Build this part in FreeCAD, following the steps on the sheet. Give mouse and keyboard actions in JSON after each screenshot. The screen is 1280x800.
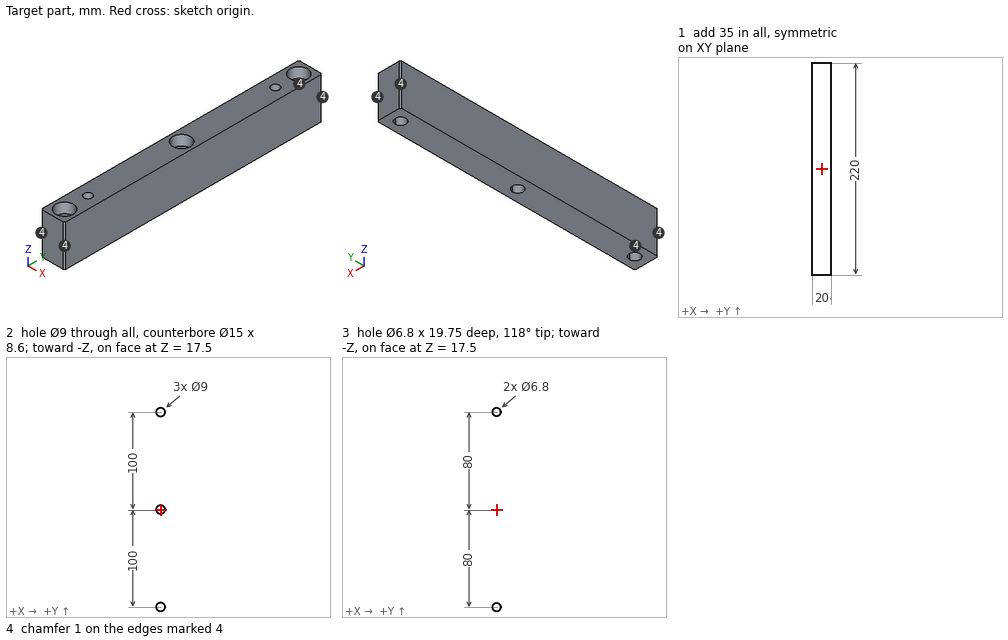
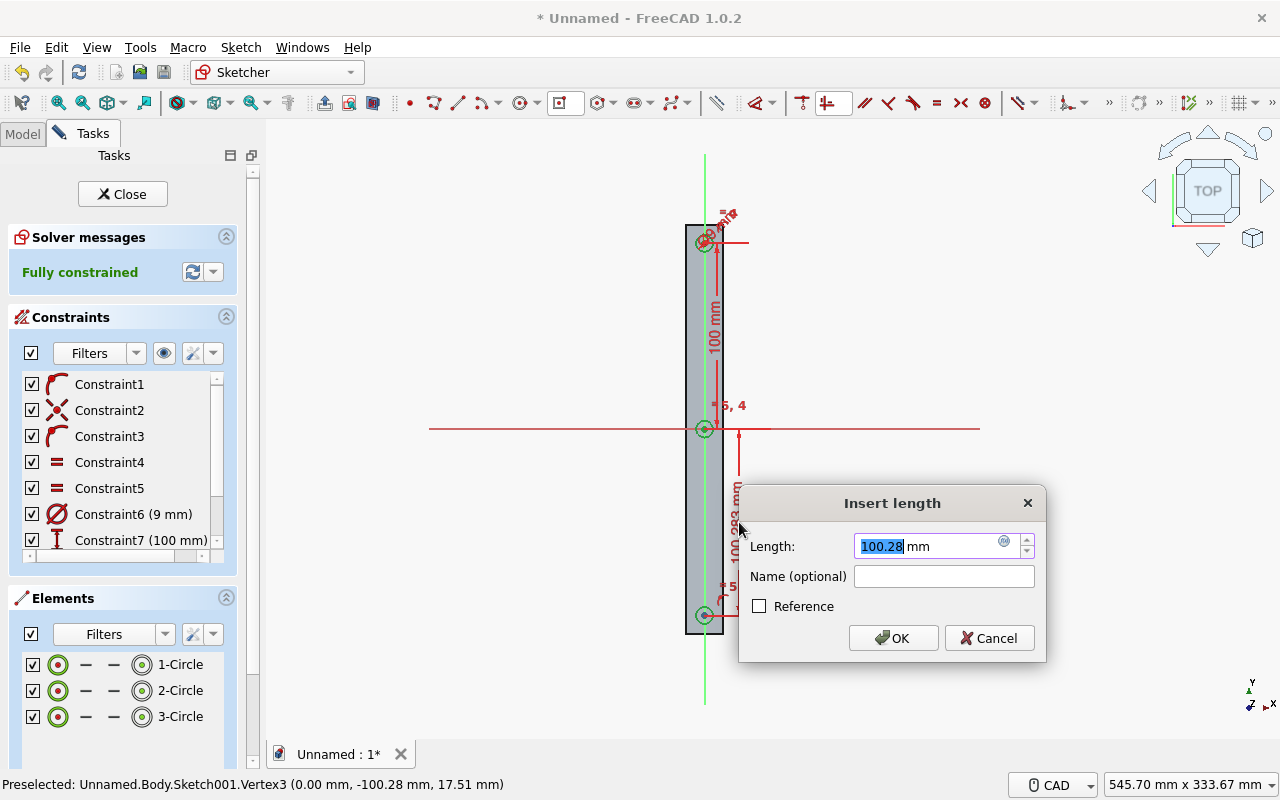
{"action": "type", "text": "100"}
{"action": "key", "text": "Return"}
{"action": "key", "text": "Escape"}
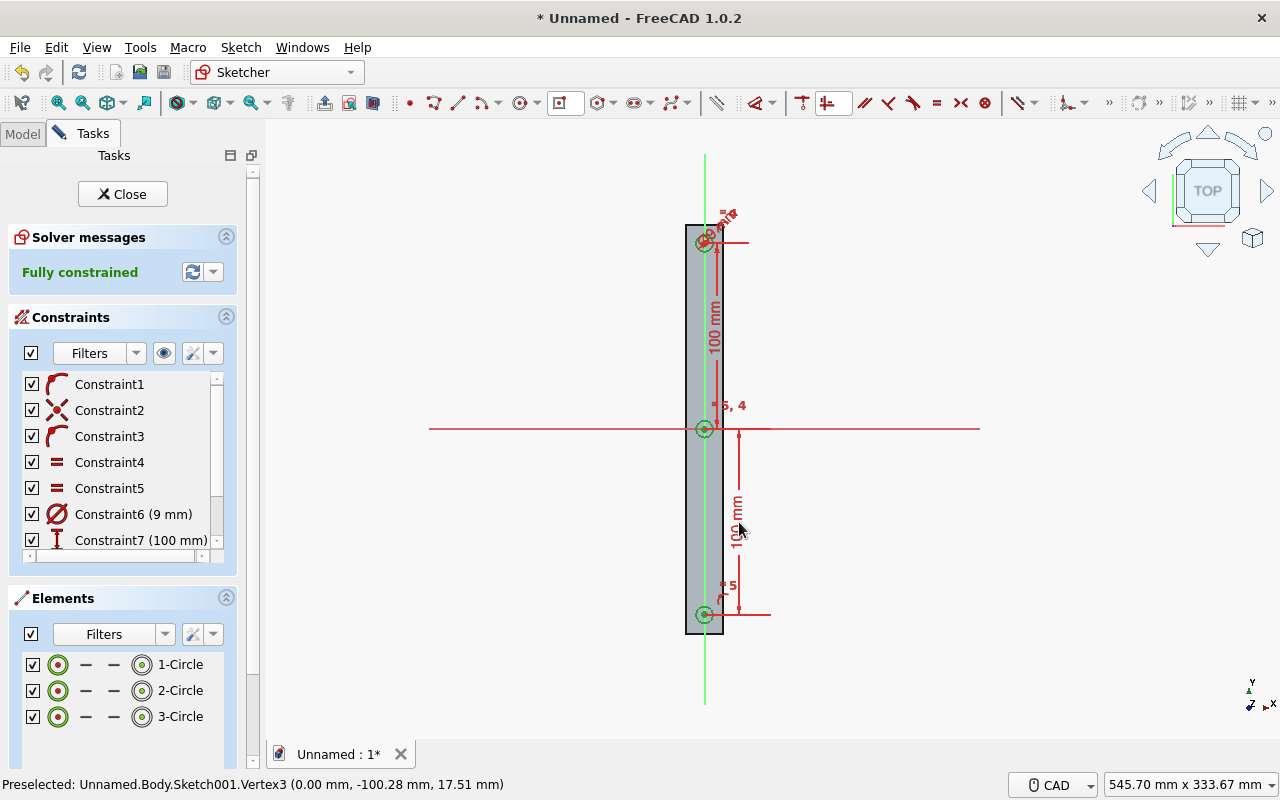
{"action": "left_click", "coordinate": [123, 194]}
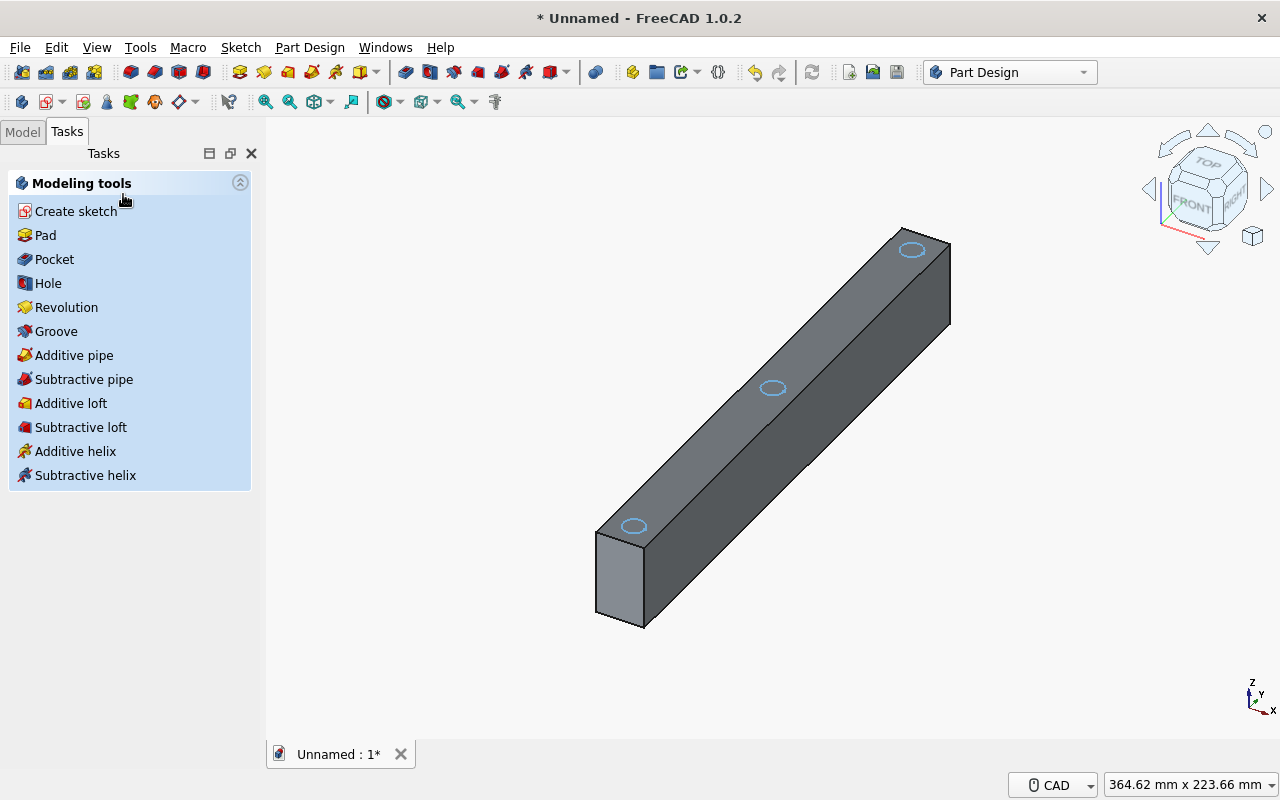
{"action": "left_click", "coordinate": [430, 72]}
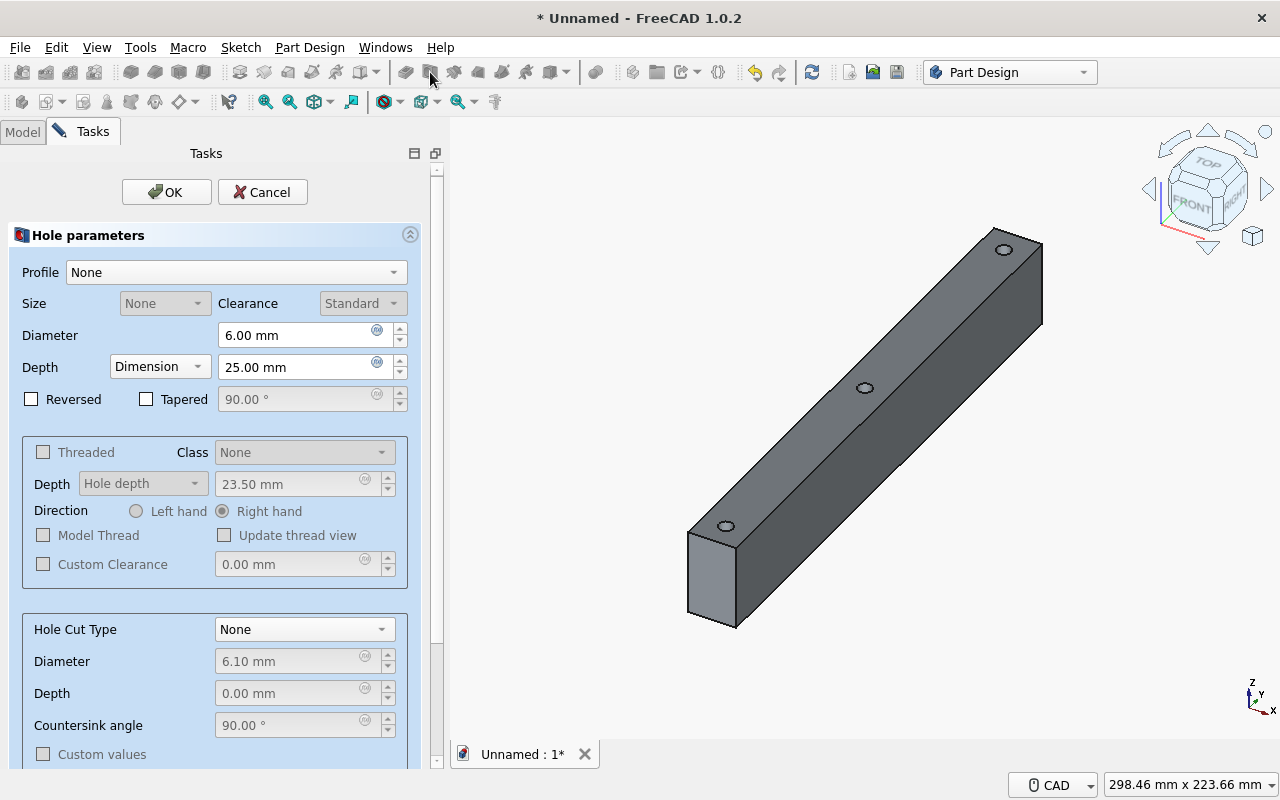
{"action": "triple_click", "coordinate": [305, 335]}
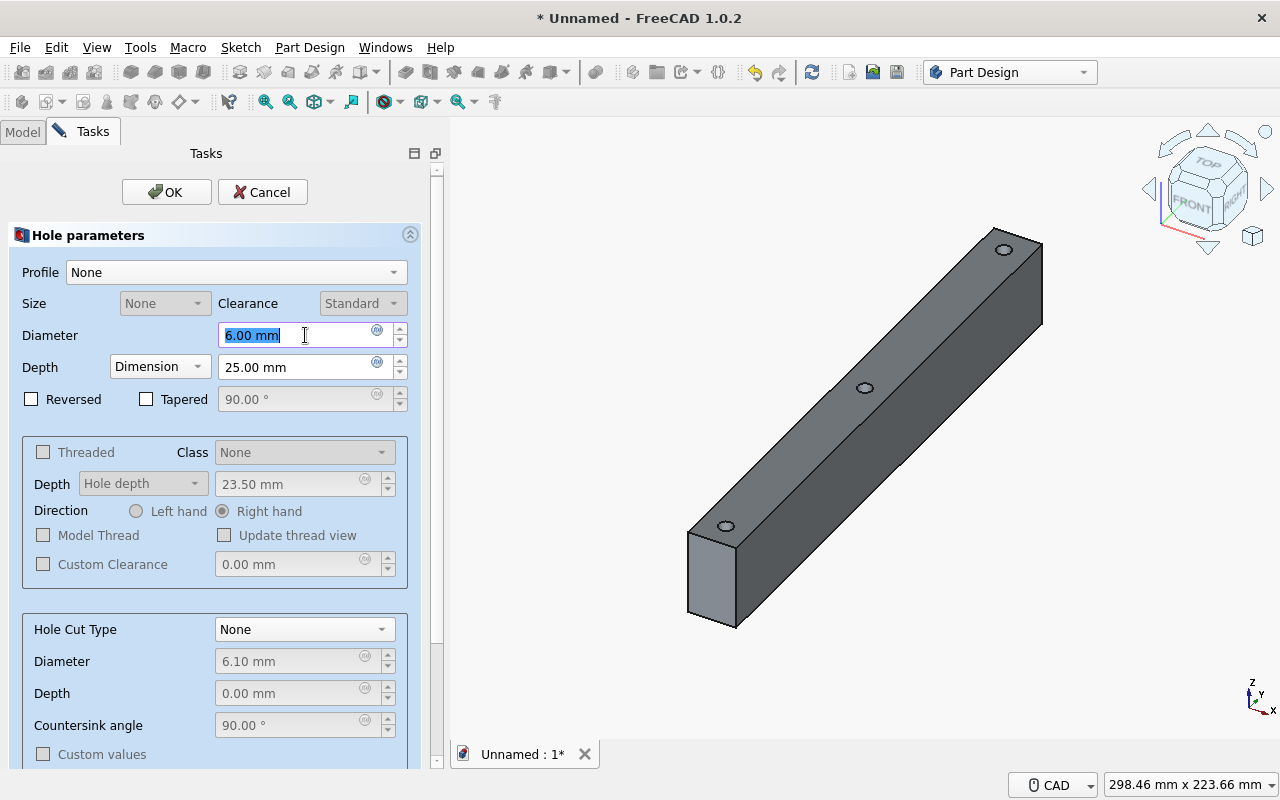
{"action": "type", "text": "9"}
{"action": "key", "text": "Tab"}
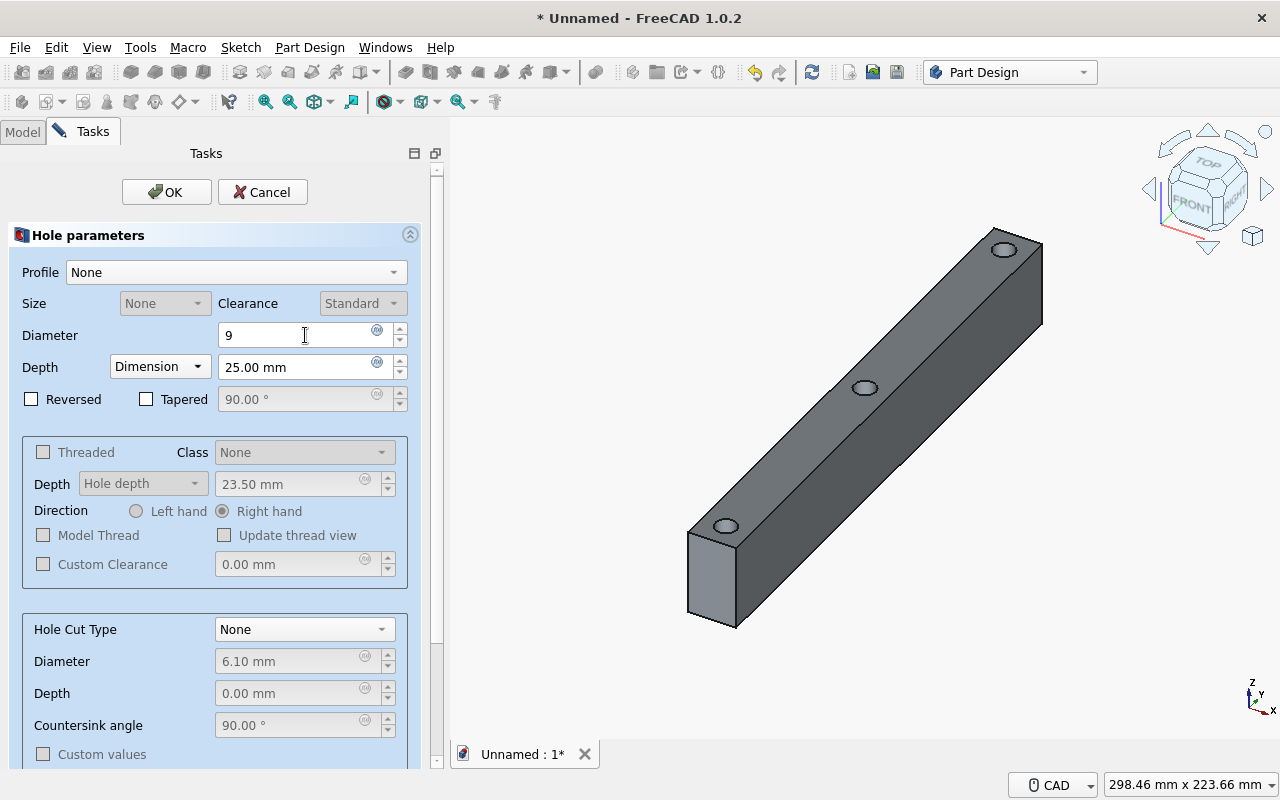
{"action": "left_click", "coordinate": [161, 366]}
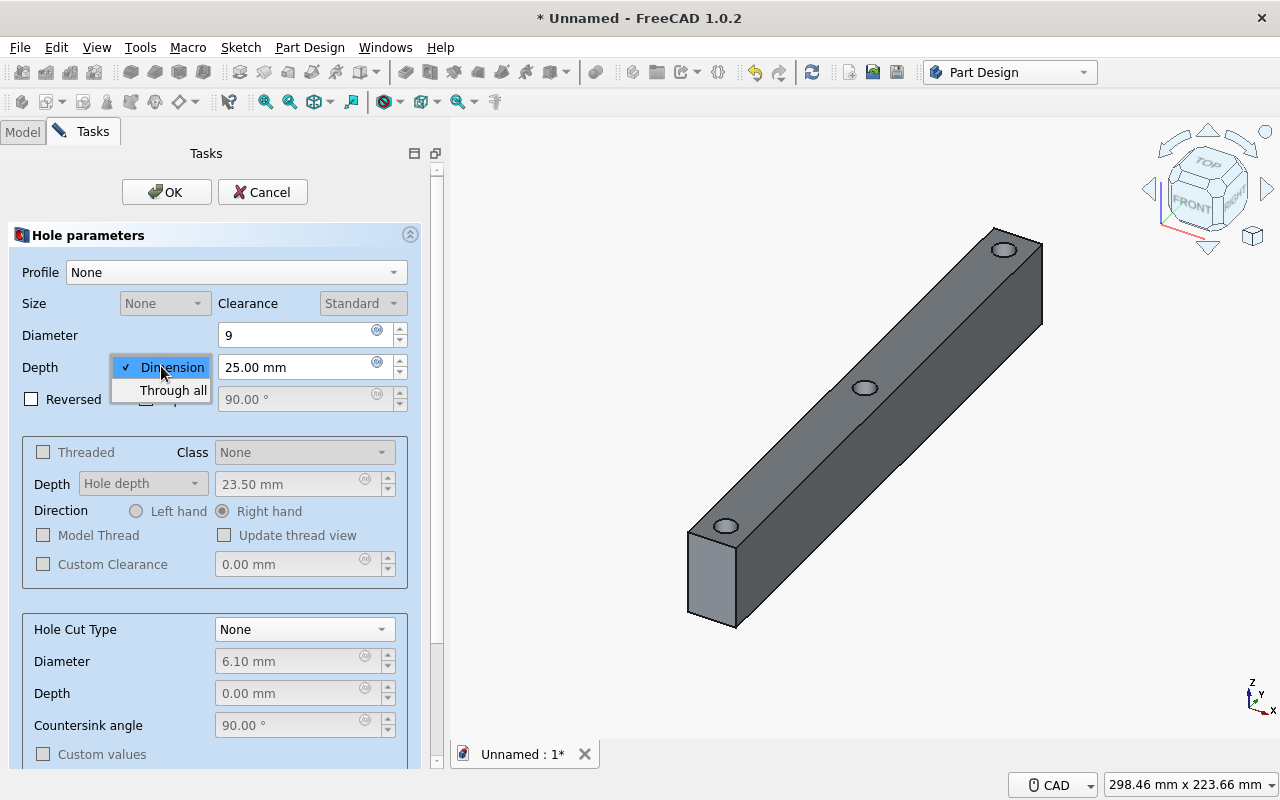
{"action": "left_click", "coordinate": [160, 390]}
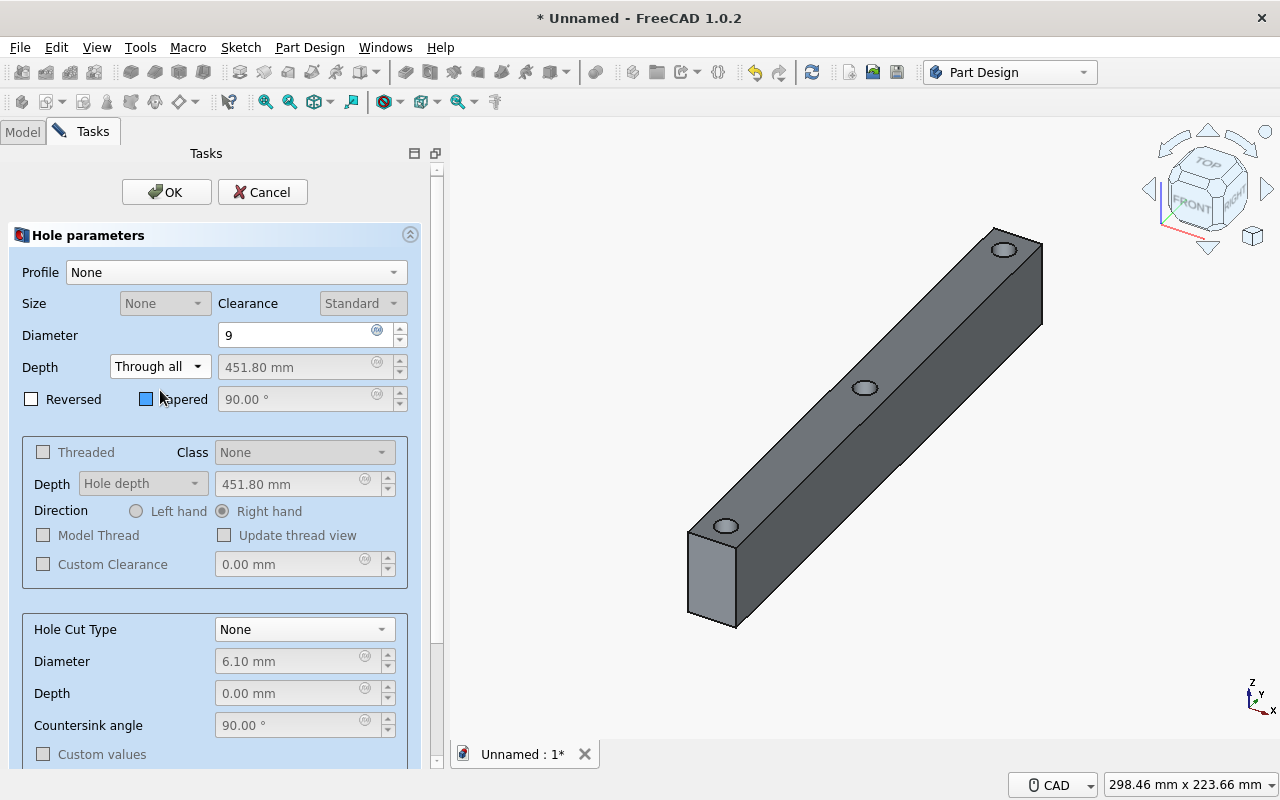
{"action": "left_click", "coordinate": [306, 630]}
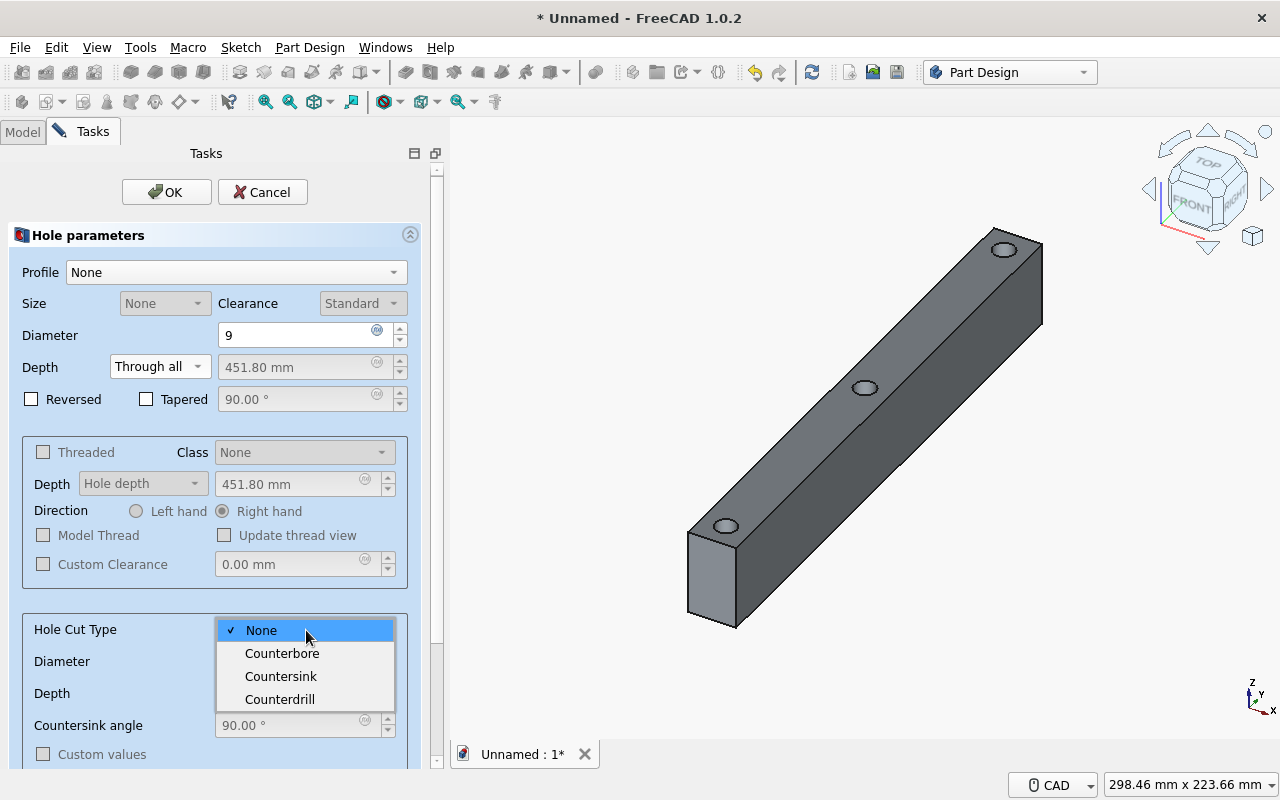
{"action": "left_click", "coordinate": [304, 654]}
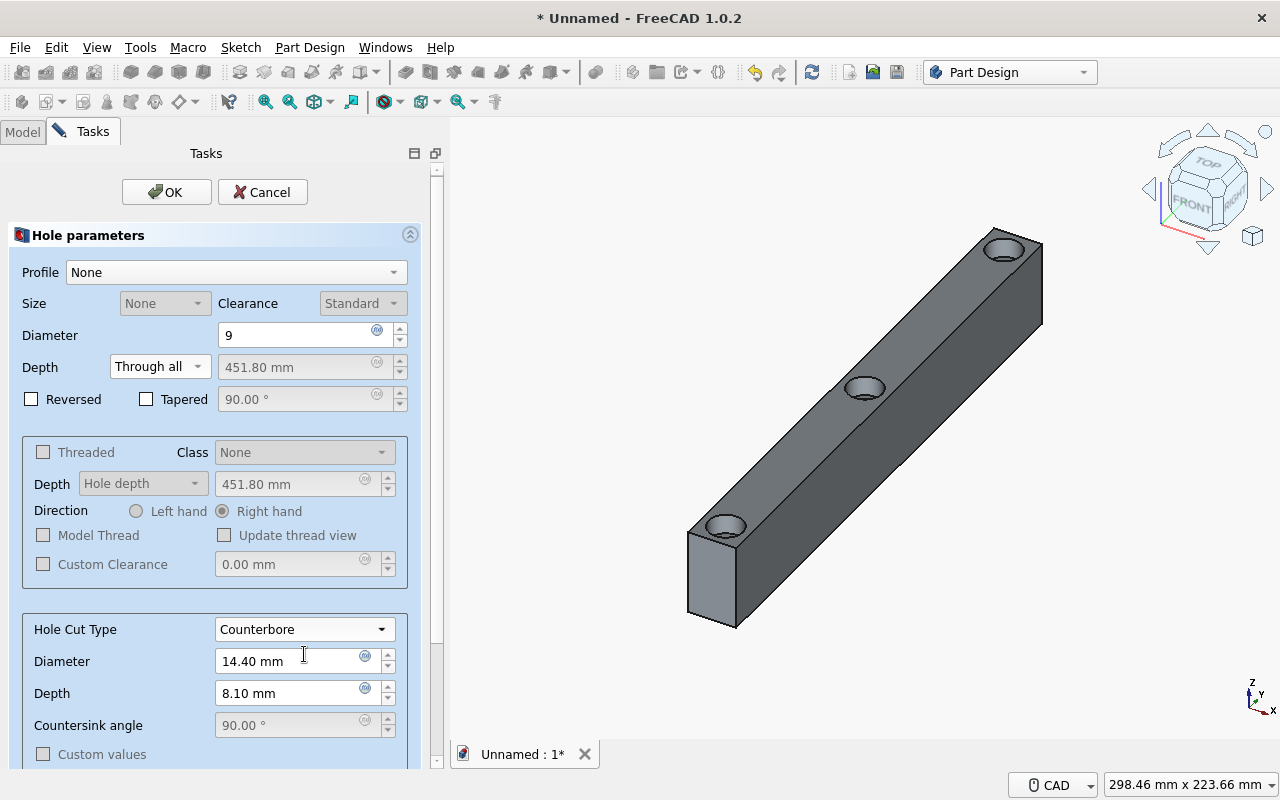
{"action": "triple_click", "coordinate": [298, 661]}